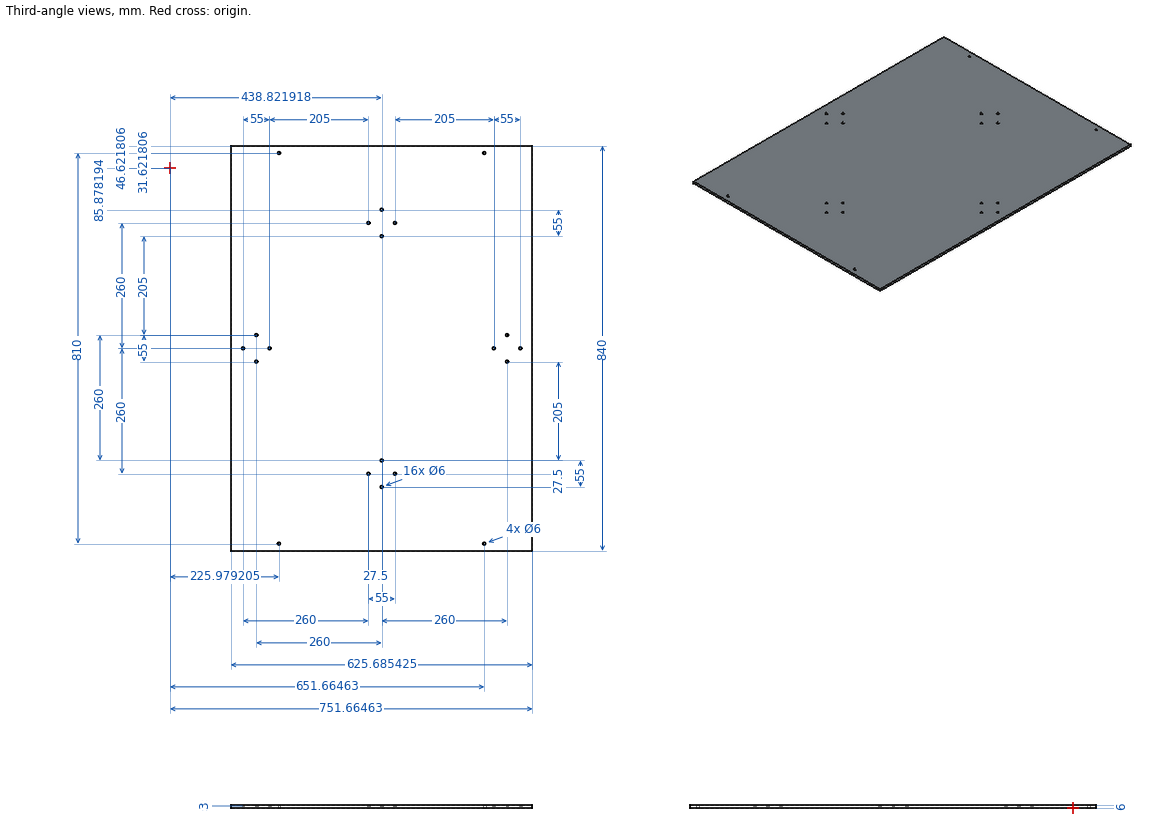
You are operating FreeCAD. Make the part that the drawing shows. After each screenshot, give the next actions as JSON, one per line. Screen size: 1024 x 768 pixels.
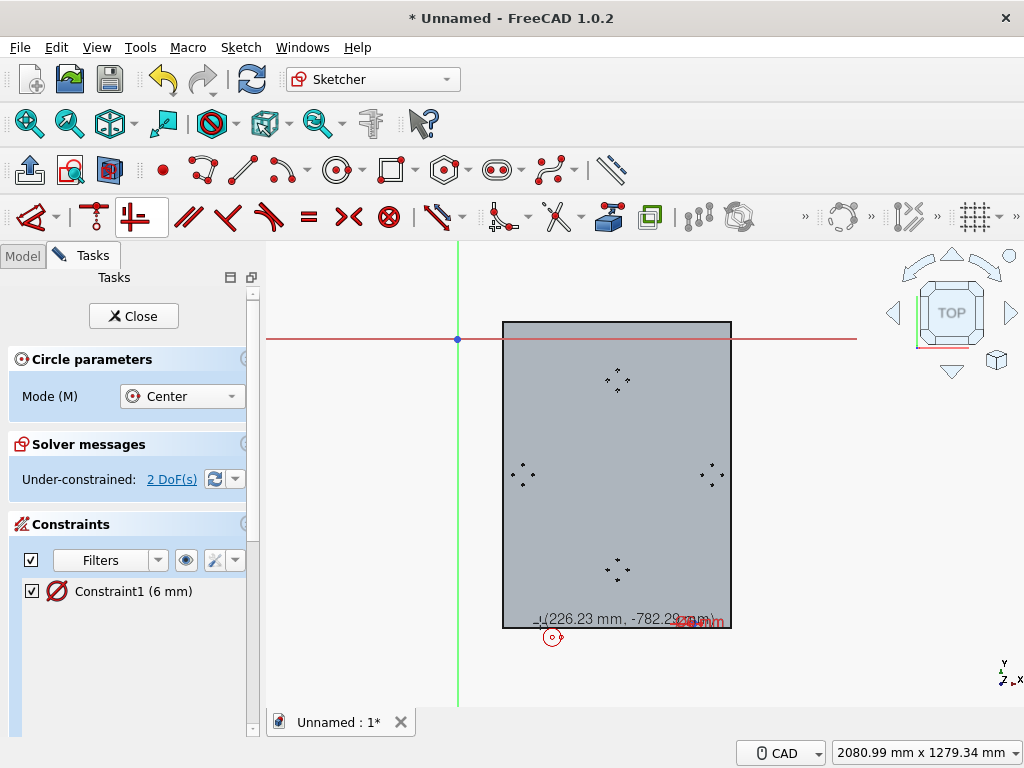
{"action": "left_click", "coordinate": [540, 623]}
{"action": "mouse_move", "coordinate": [541, 622]}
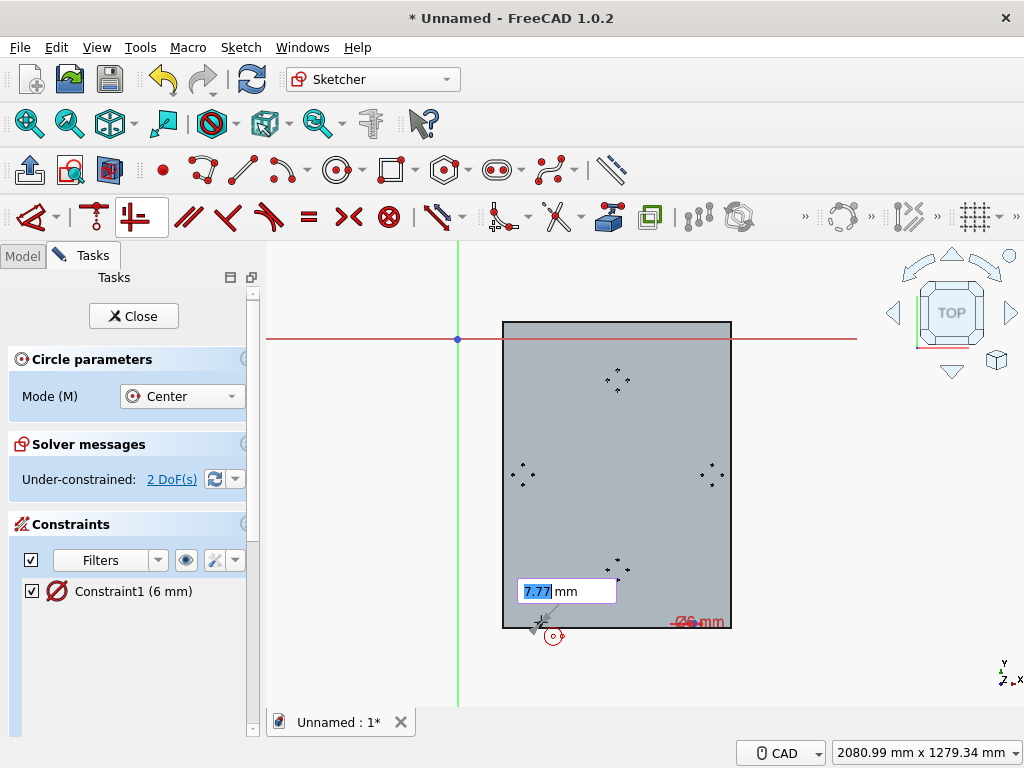
{"action": "type", "text": "6"}
{"action": "key", "text": "Return"}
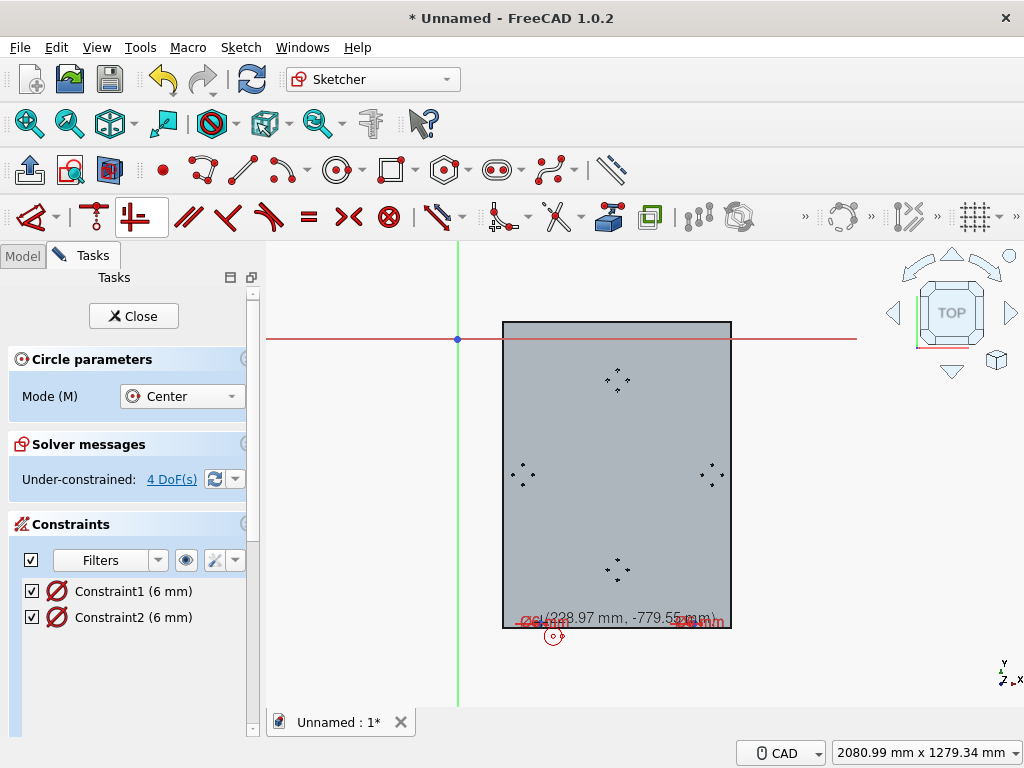
{"action": "scroll", "coordinate": [540, 328], "scroll_direction": "up", "scroll_amount": 16}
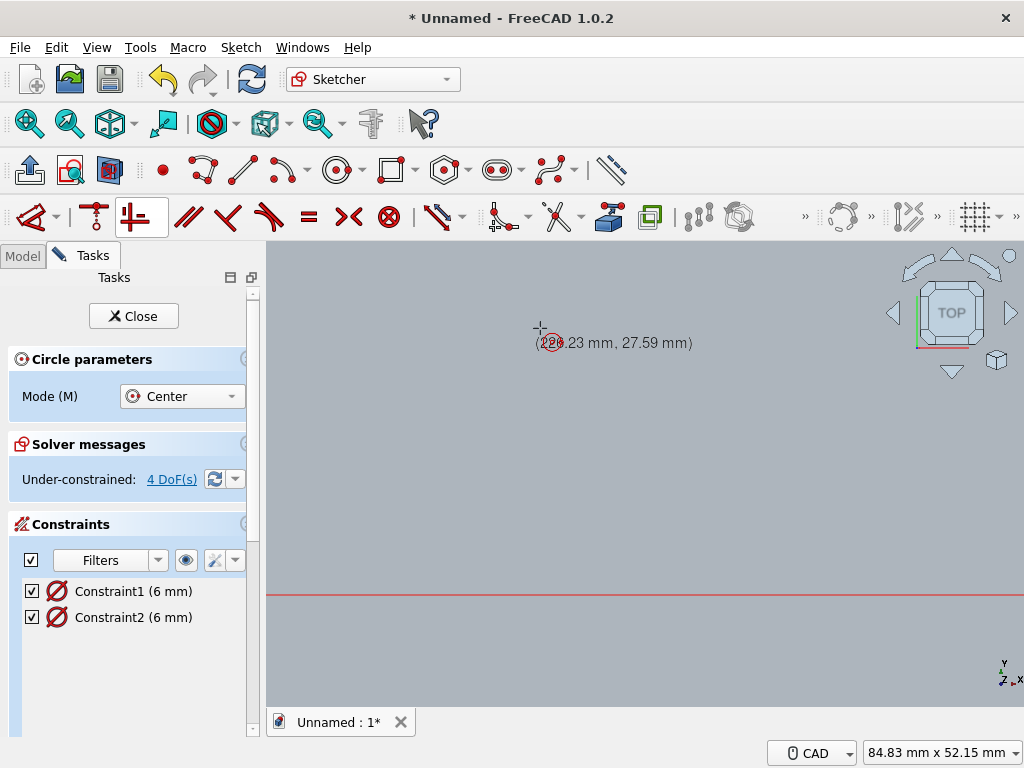
{"action": "scroll", "coordinate": [540, 327], "scroll_direction": "down", "scroll_amount": 16}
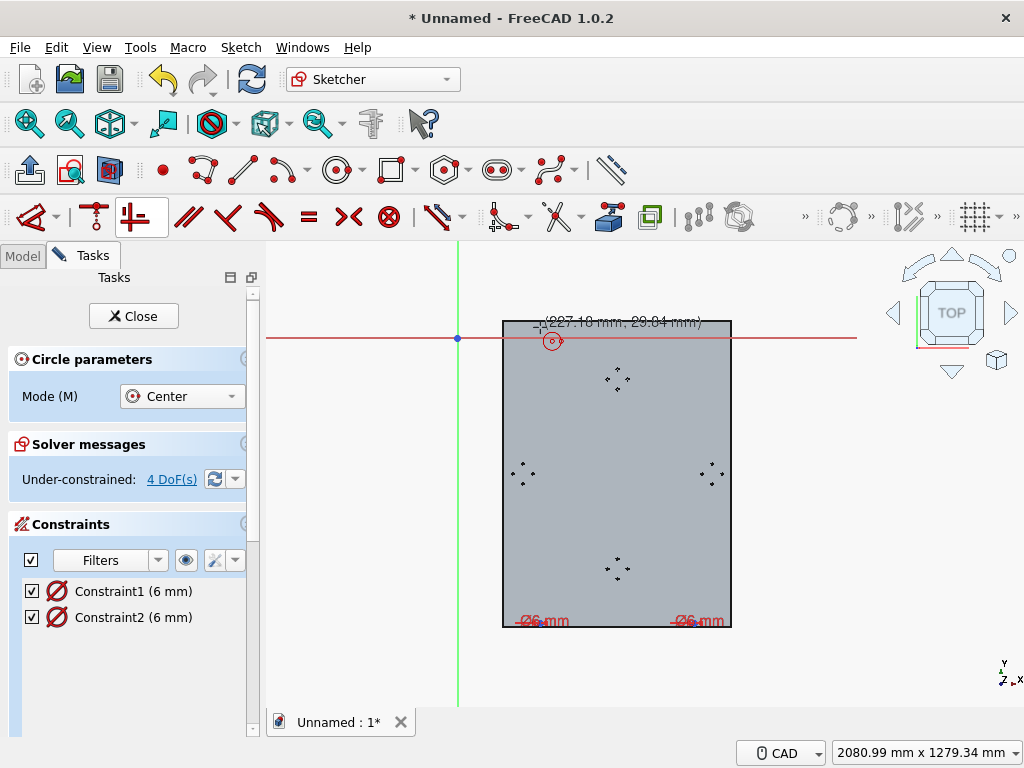
{"action": "scroll", "coordinate": [540, 327], "scroll_direction": "up", "scroll_amount": 2}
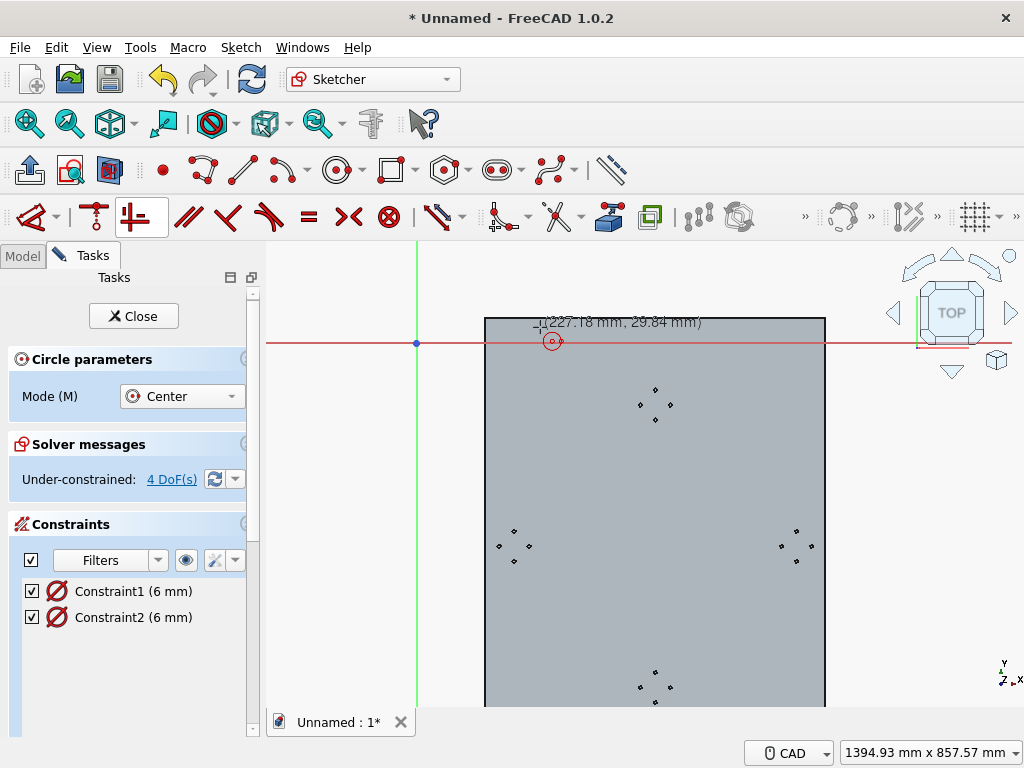
{"action": "left_click", "coordinate": [540, 326]}
{"action": "mouse_move", "coordinate": [541, 325]}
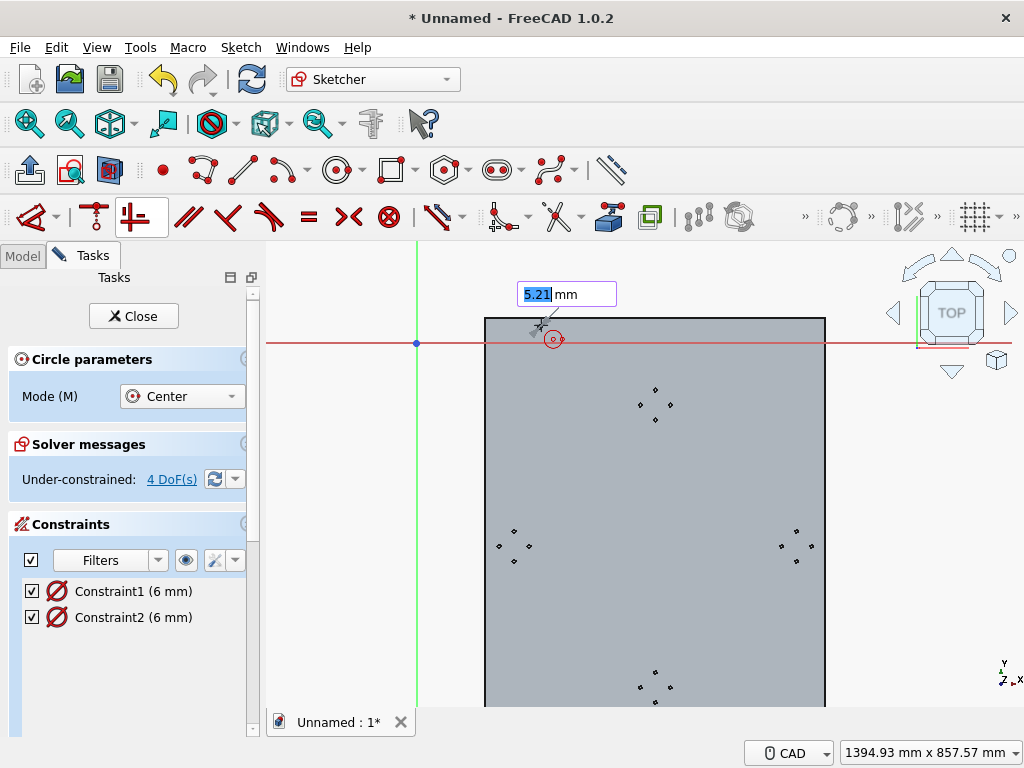
{"action": "type", "text": "6"}
{"action": "key", "text": "Return"}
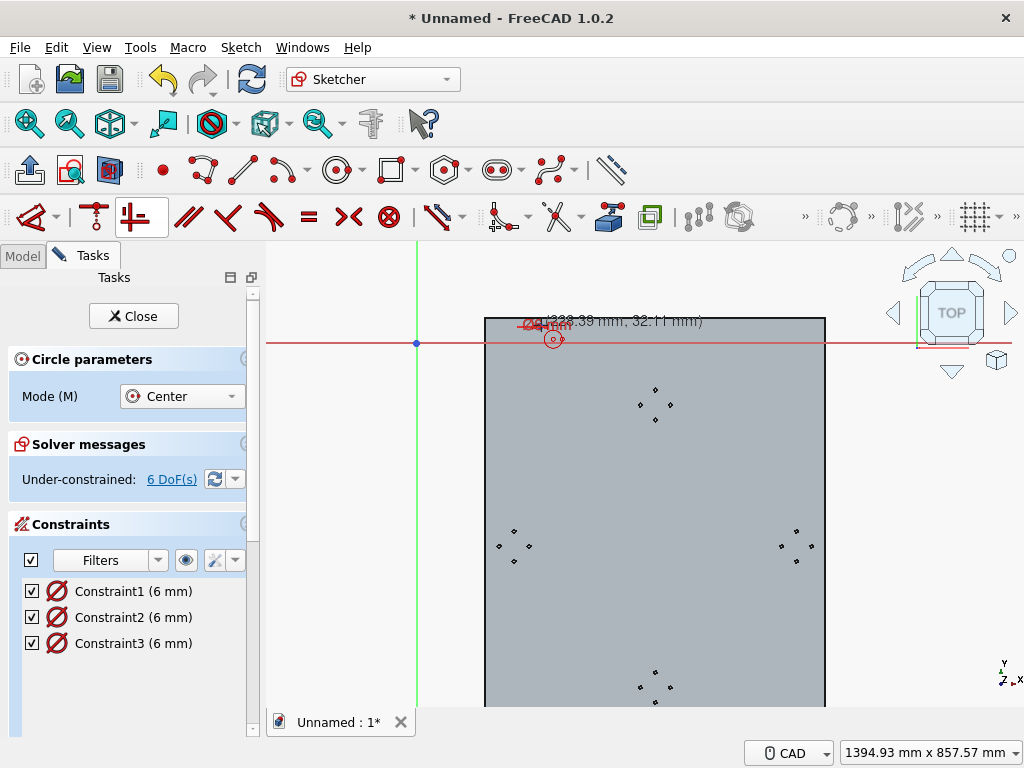
{"action": "scroll", "coordinate": [771, 326], "scroll_direction": "up", "scroll_amount": 14}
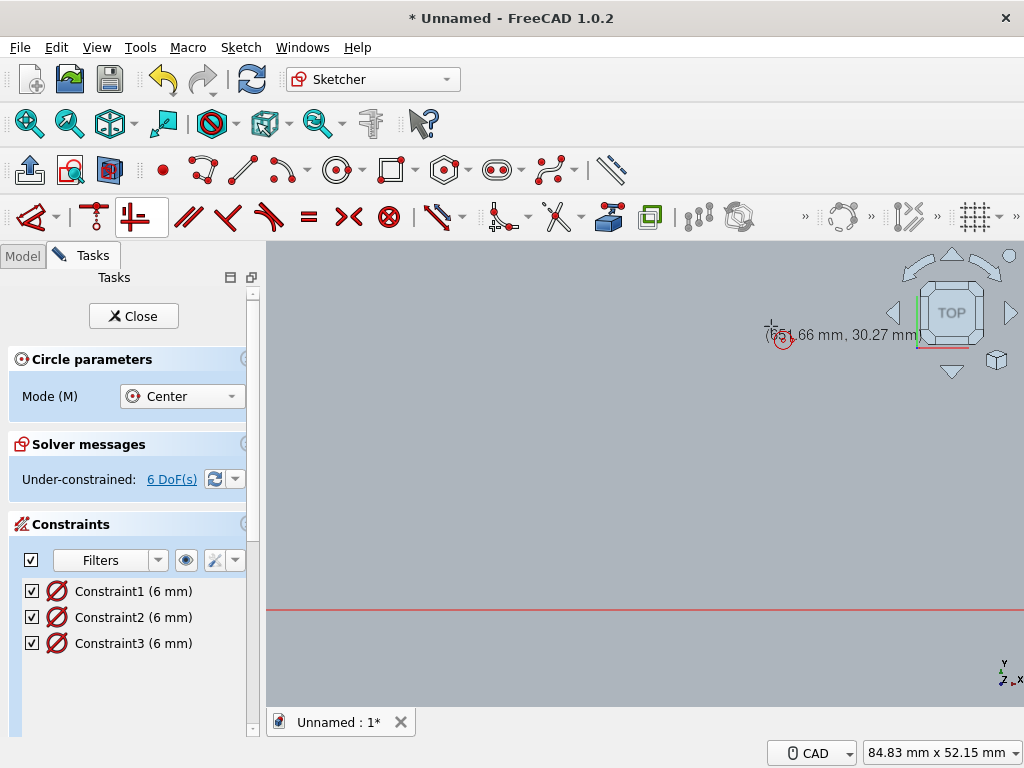
{"action": "scroll", "coordinate": [692, 326], "scroll_direction": "down", "scroll_amount": 16}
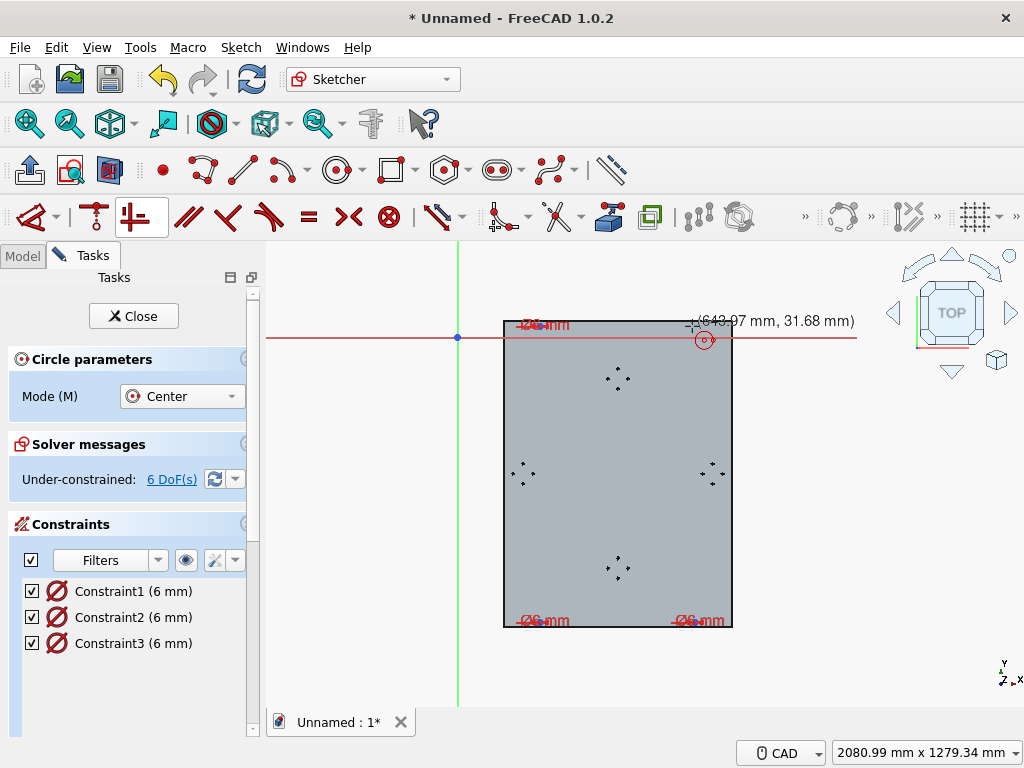
{"action": "scroll", "coordinate": [695, 326], "scroll_direction": "up", "scroll_amount": 2}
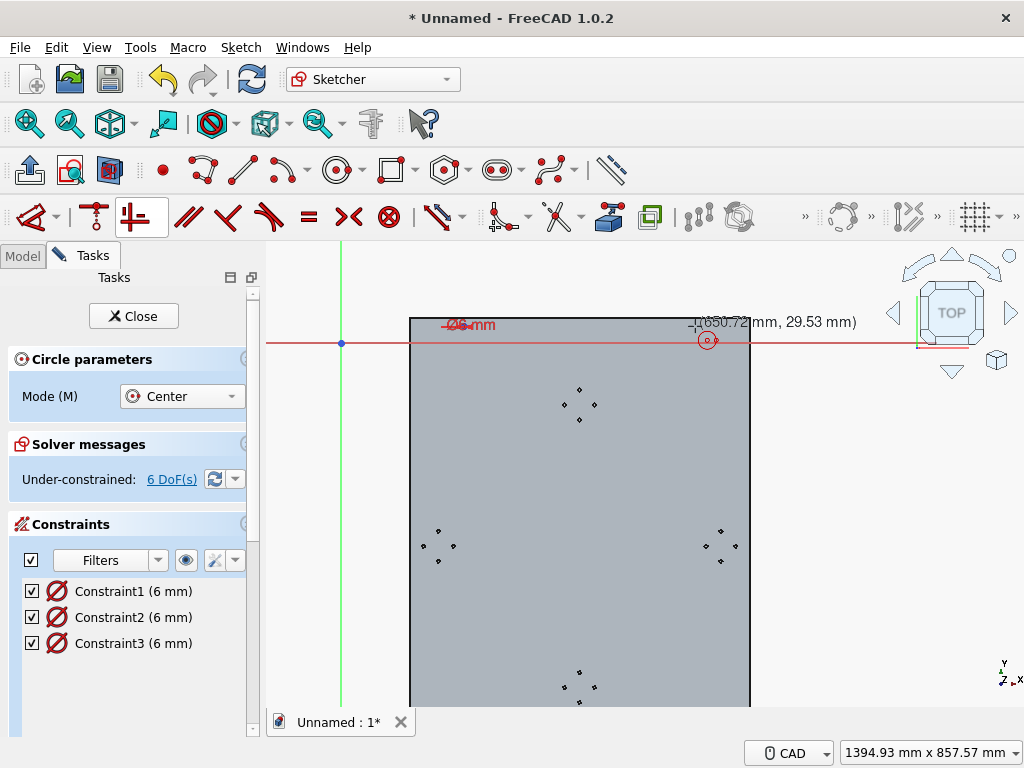
{"action": "left_click", "coordinate": [695, 326]}
{"action": "mouse_move", "coordinate": [696, 325]}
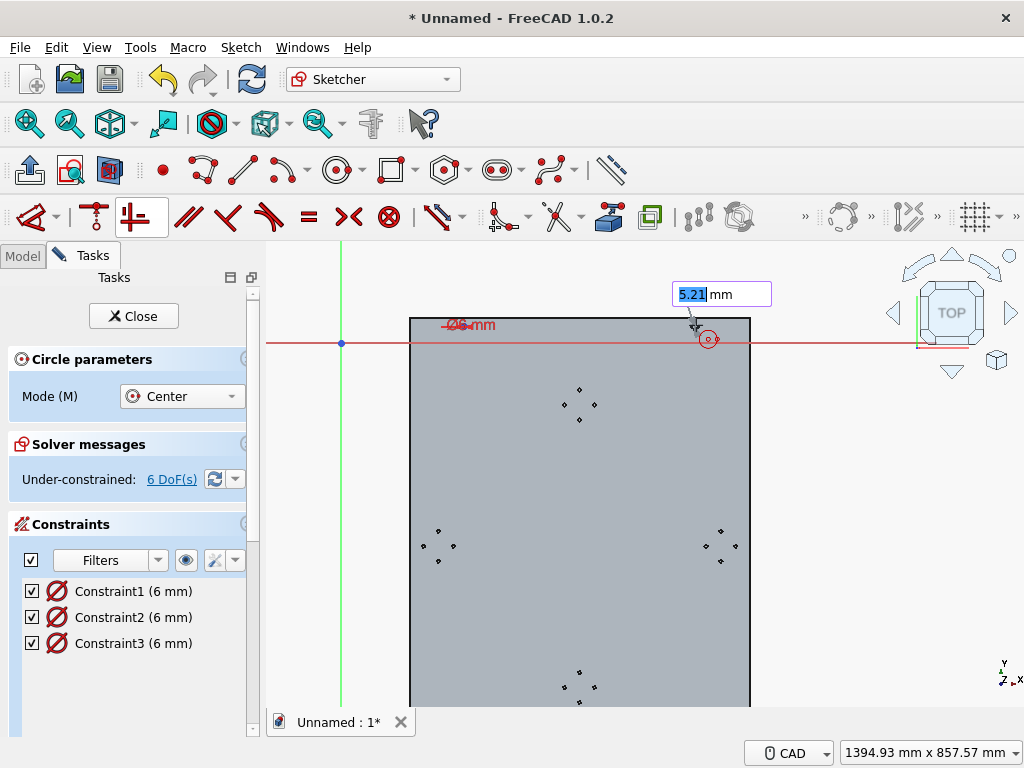
{"action": "type", "text": "6"}
{"action": "key", "text": "Return"}
{"action": "key", "text": "Escape"}